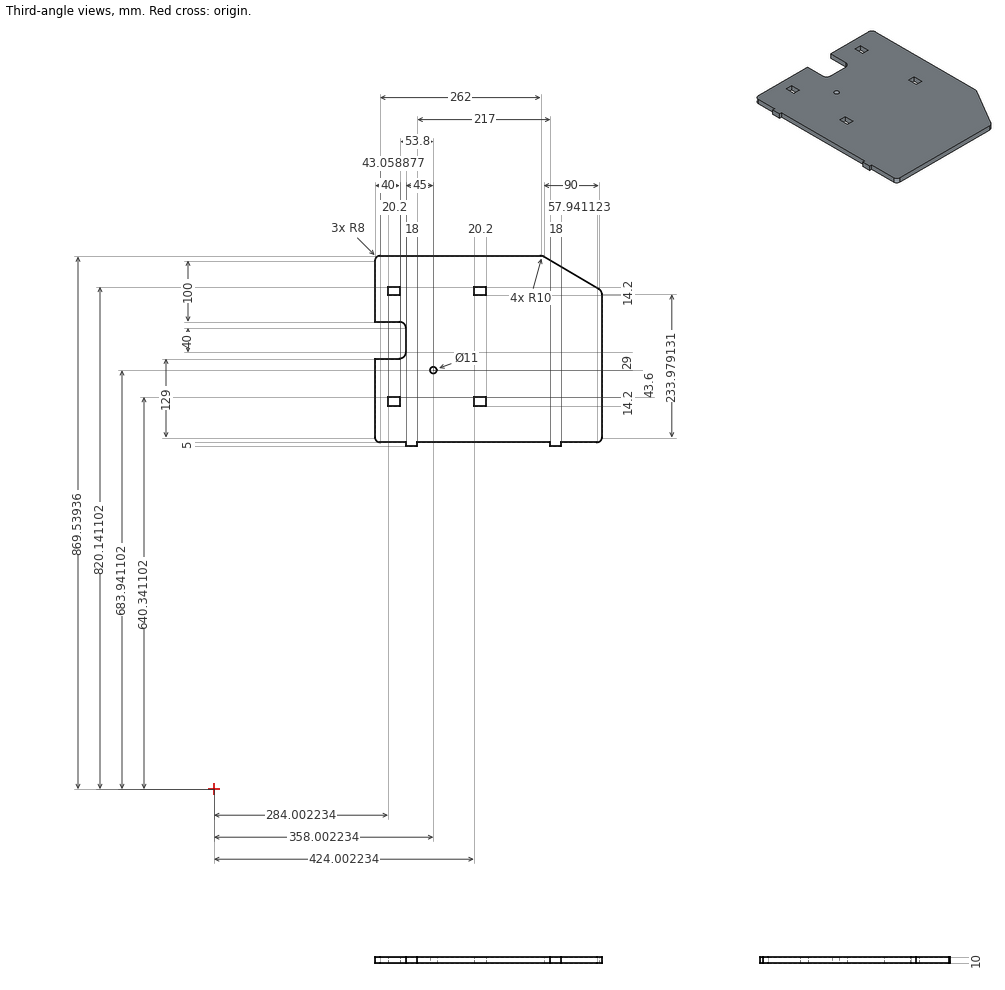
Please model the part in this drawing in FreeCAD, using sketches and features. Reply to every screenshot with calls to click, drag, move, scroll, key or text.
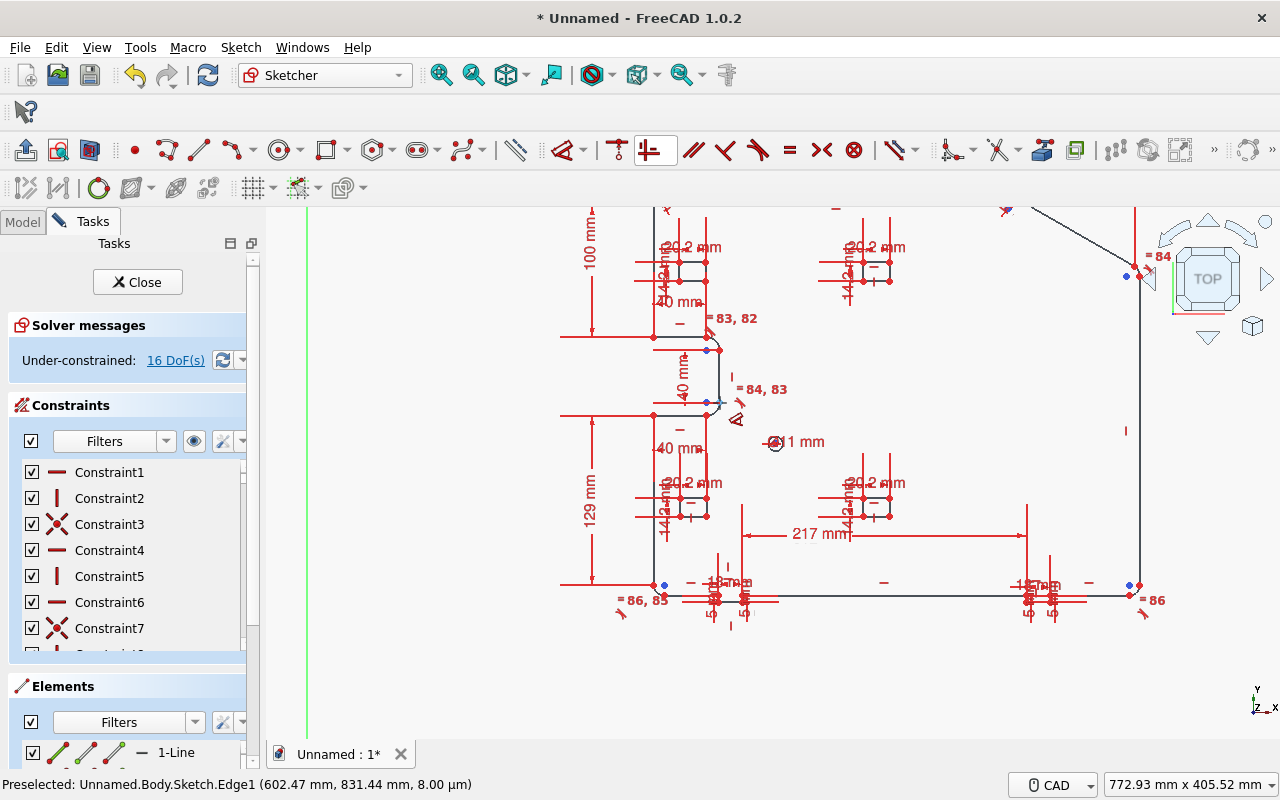
click(719, 403)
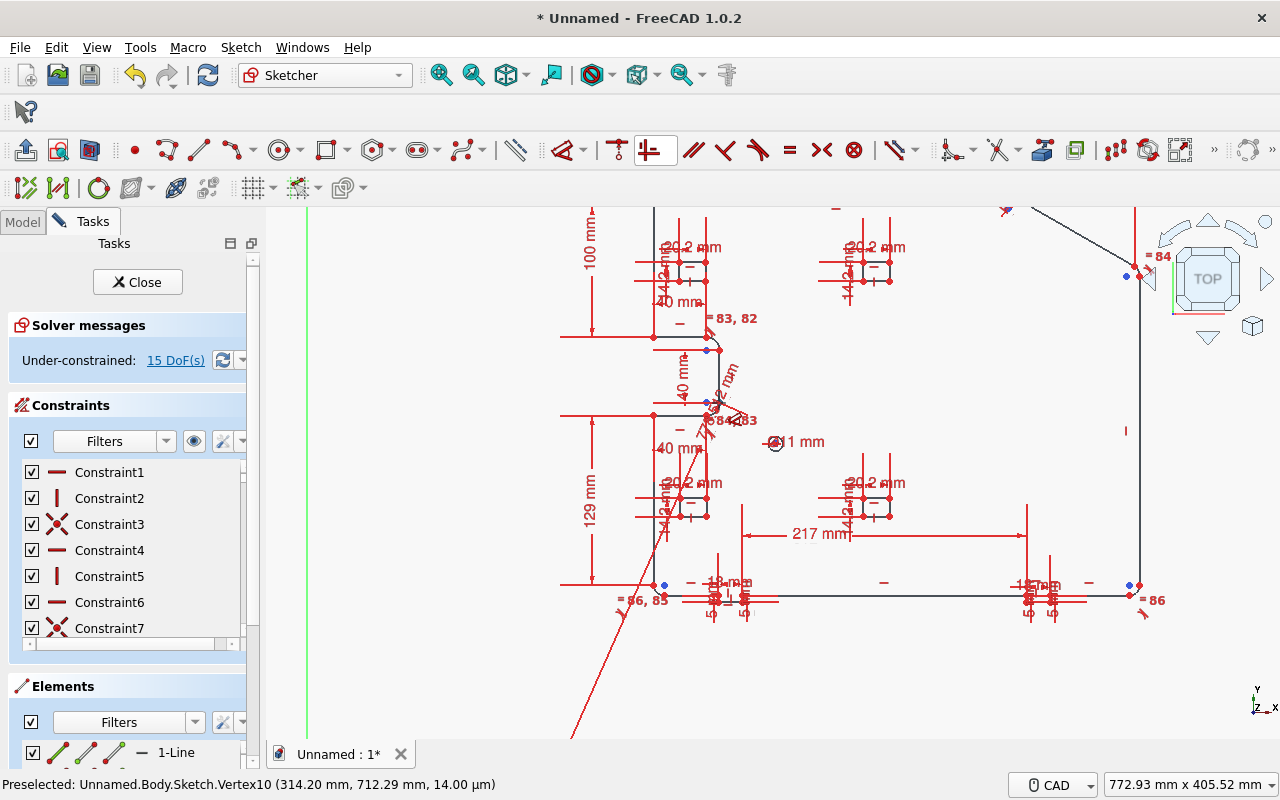
click(776, 444)
click(760, 369)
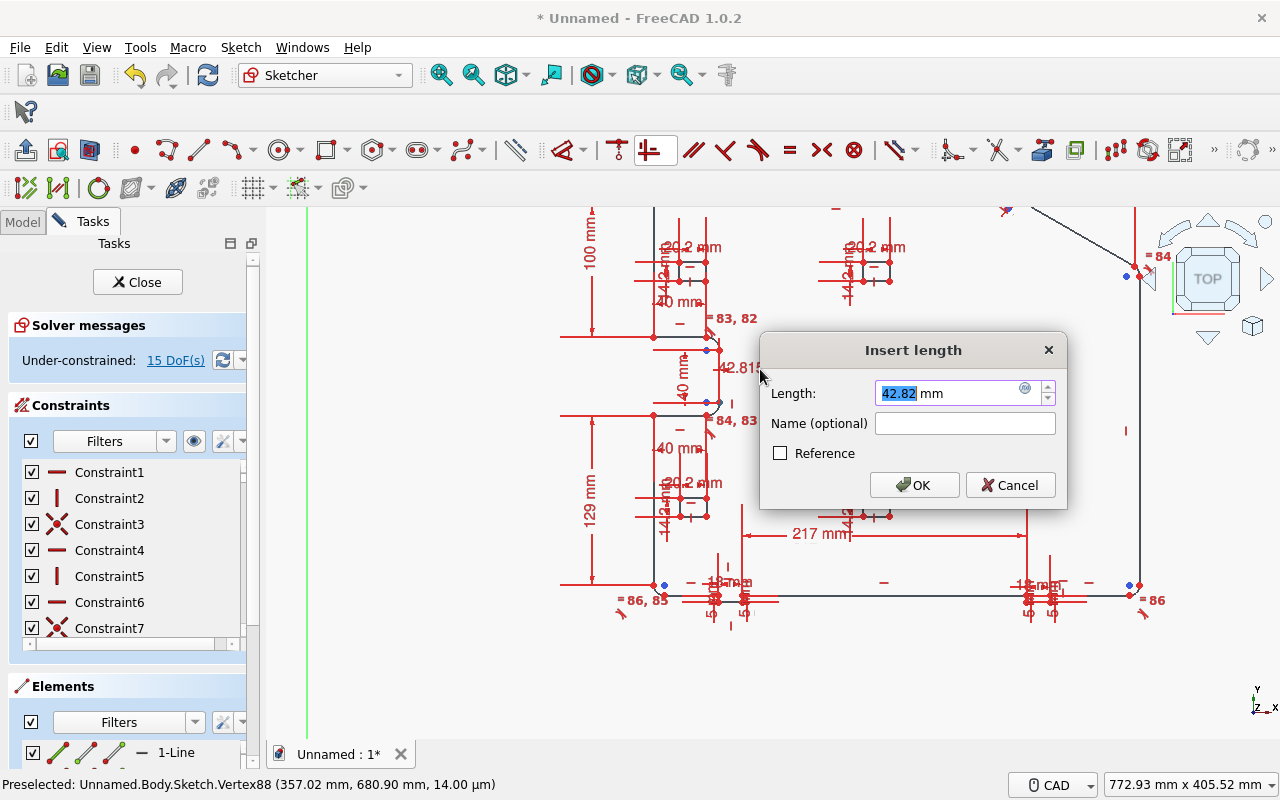
text(45)
key(Return)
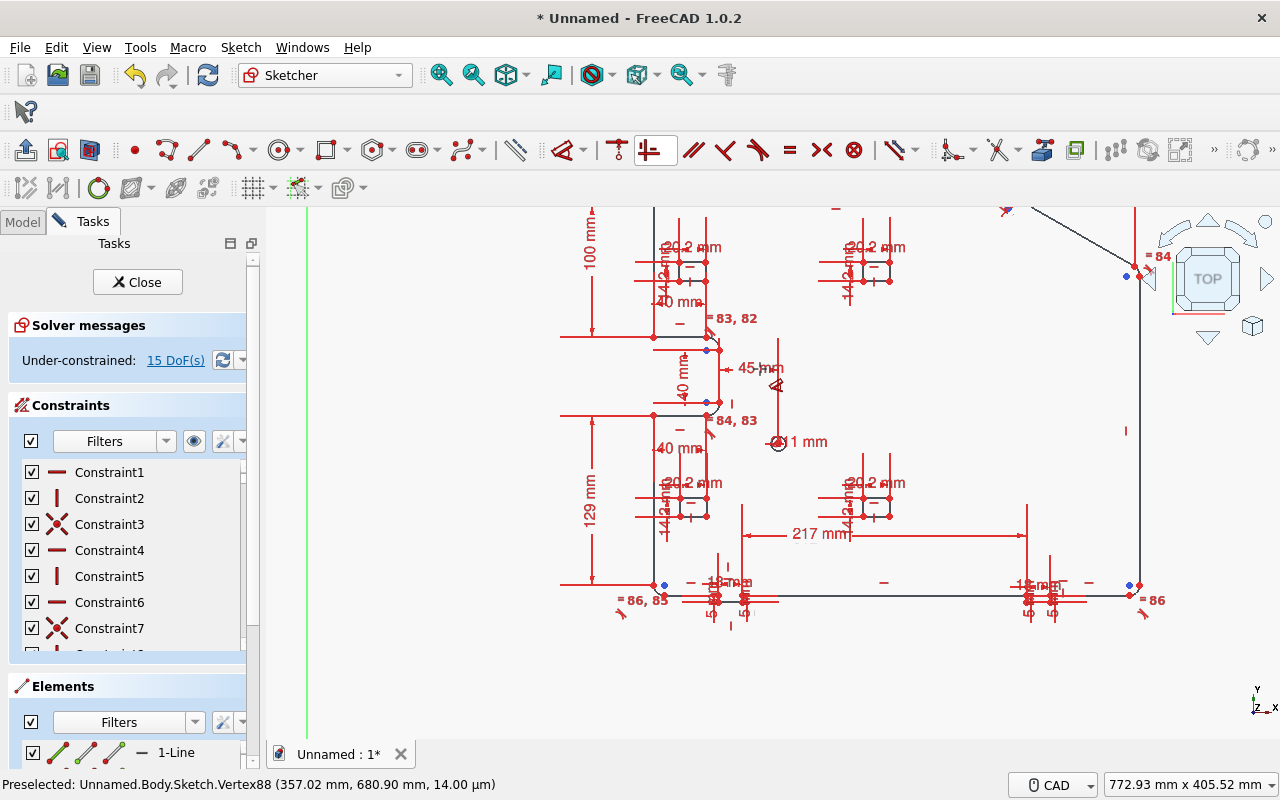
click(719, 403)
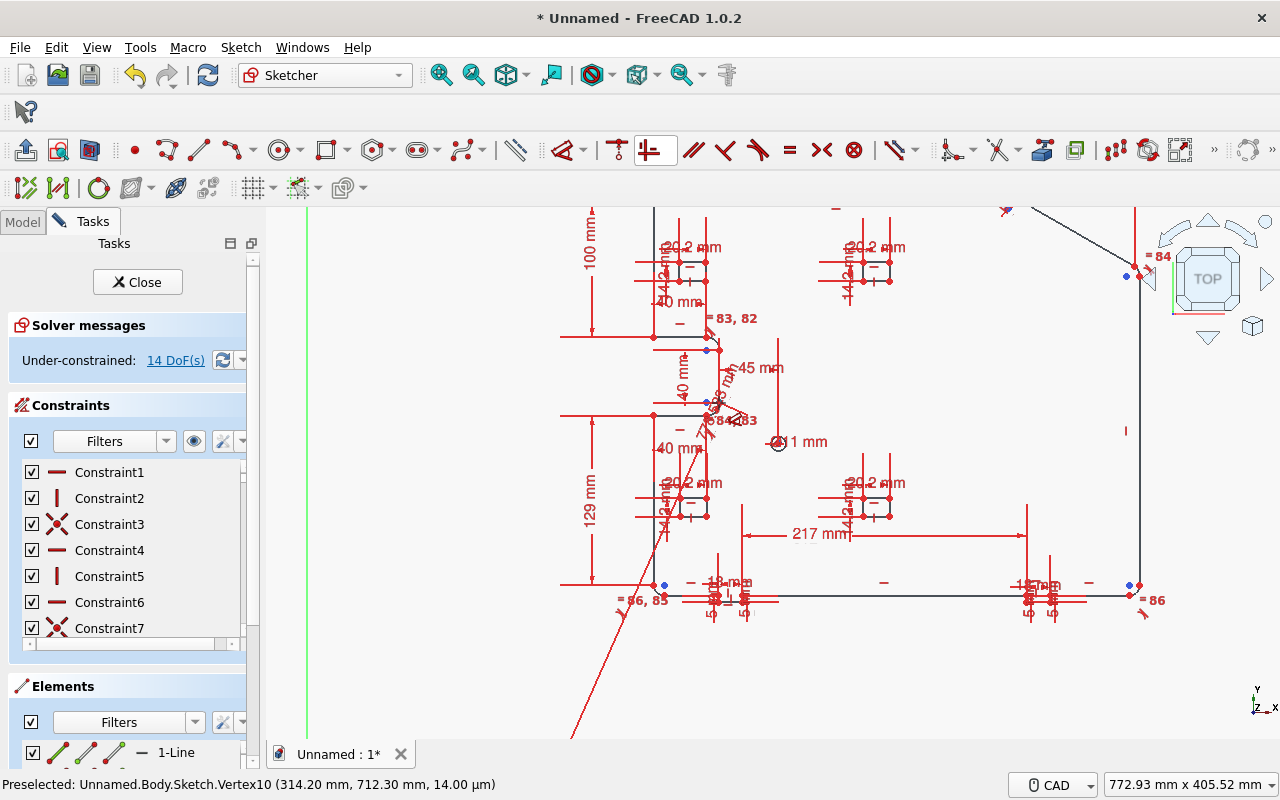
click(778, 444)
click(812, 423)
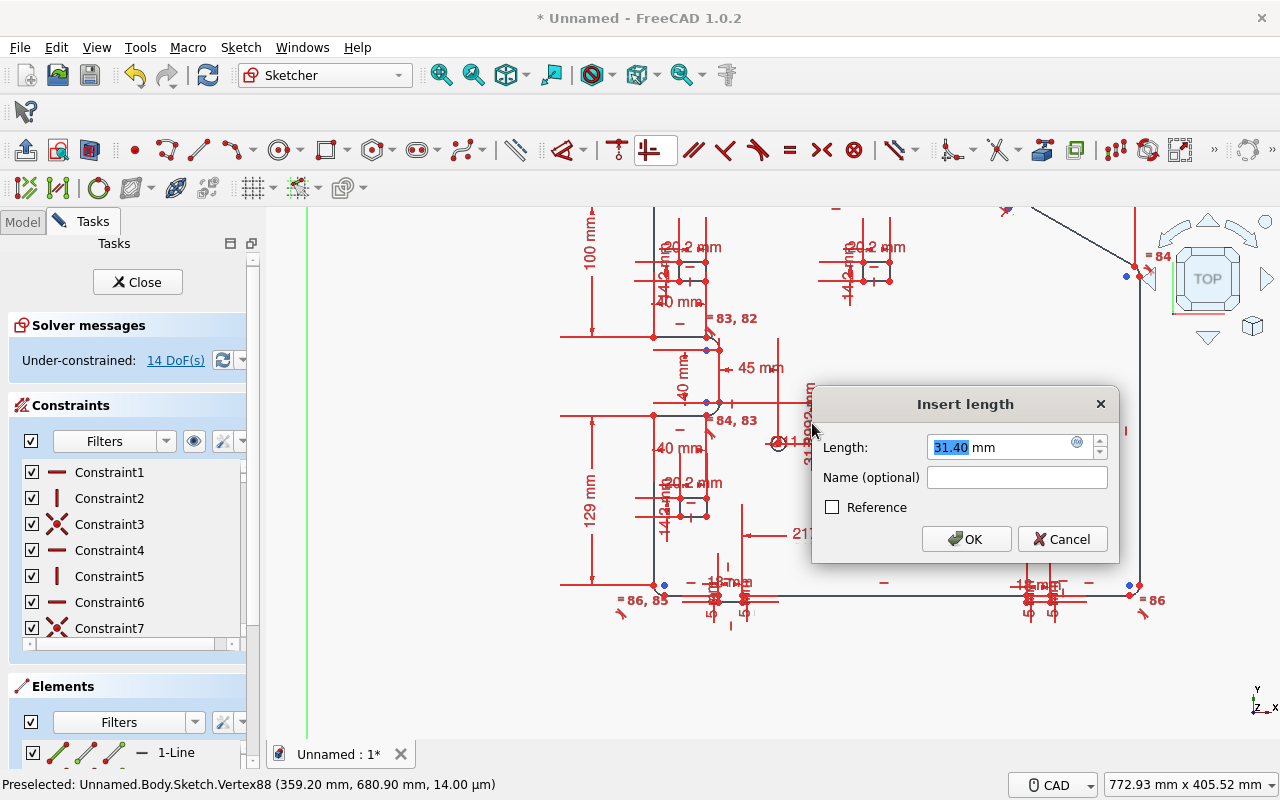
text(29)
key(Return)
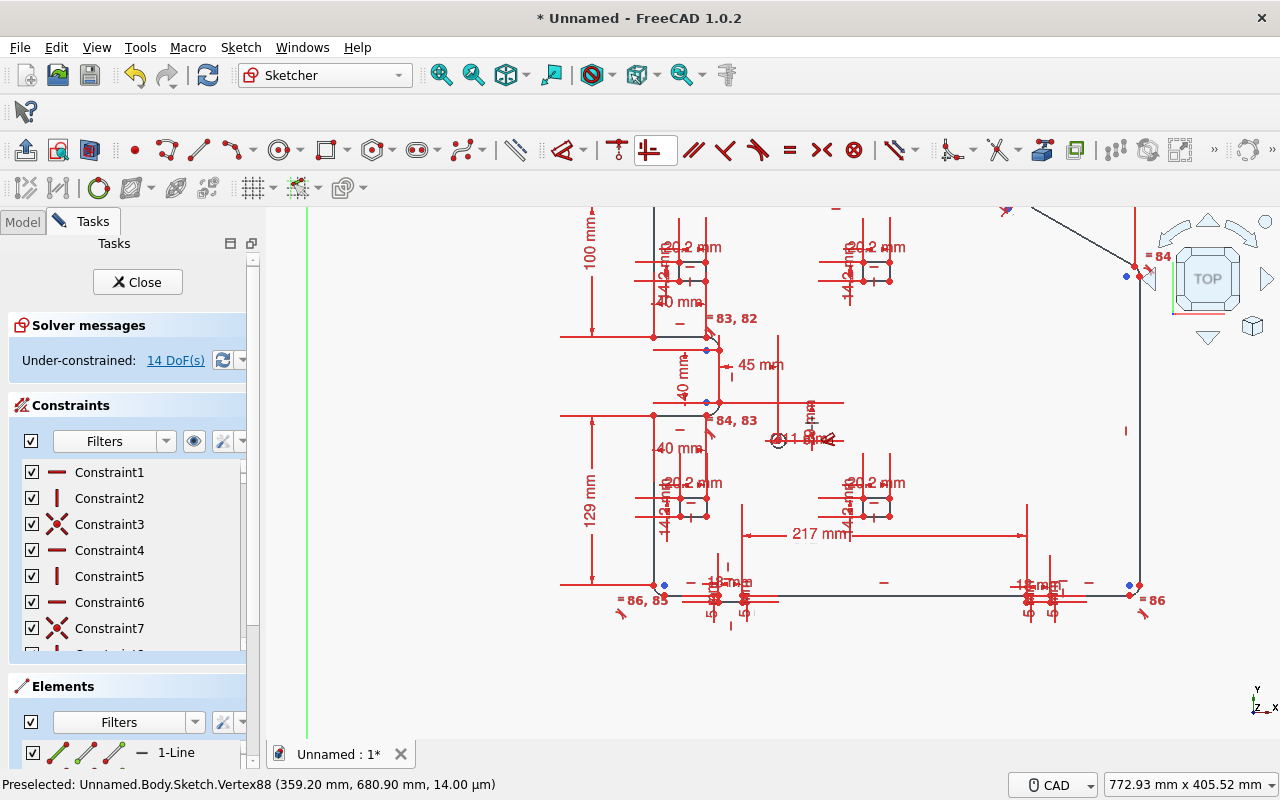
click(707, 498)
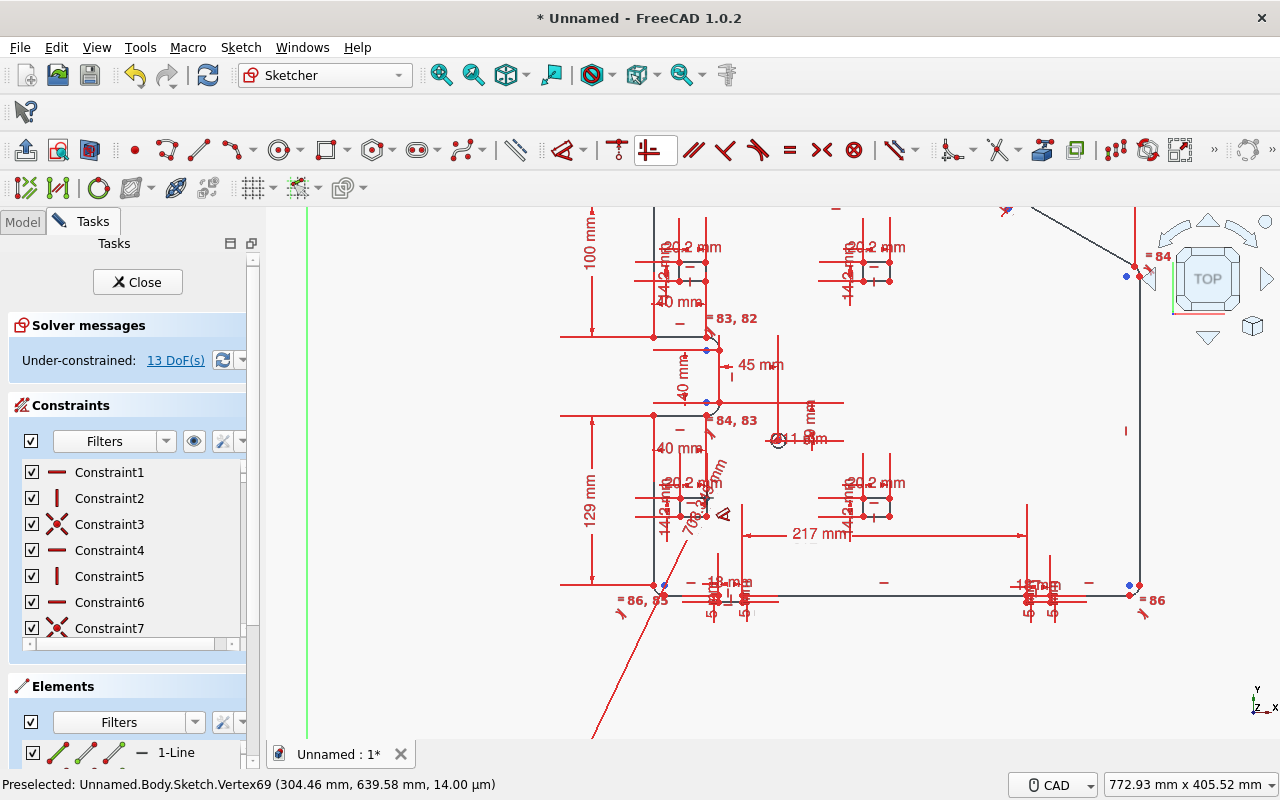
click(778, 441)
click(743, 532)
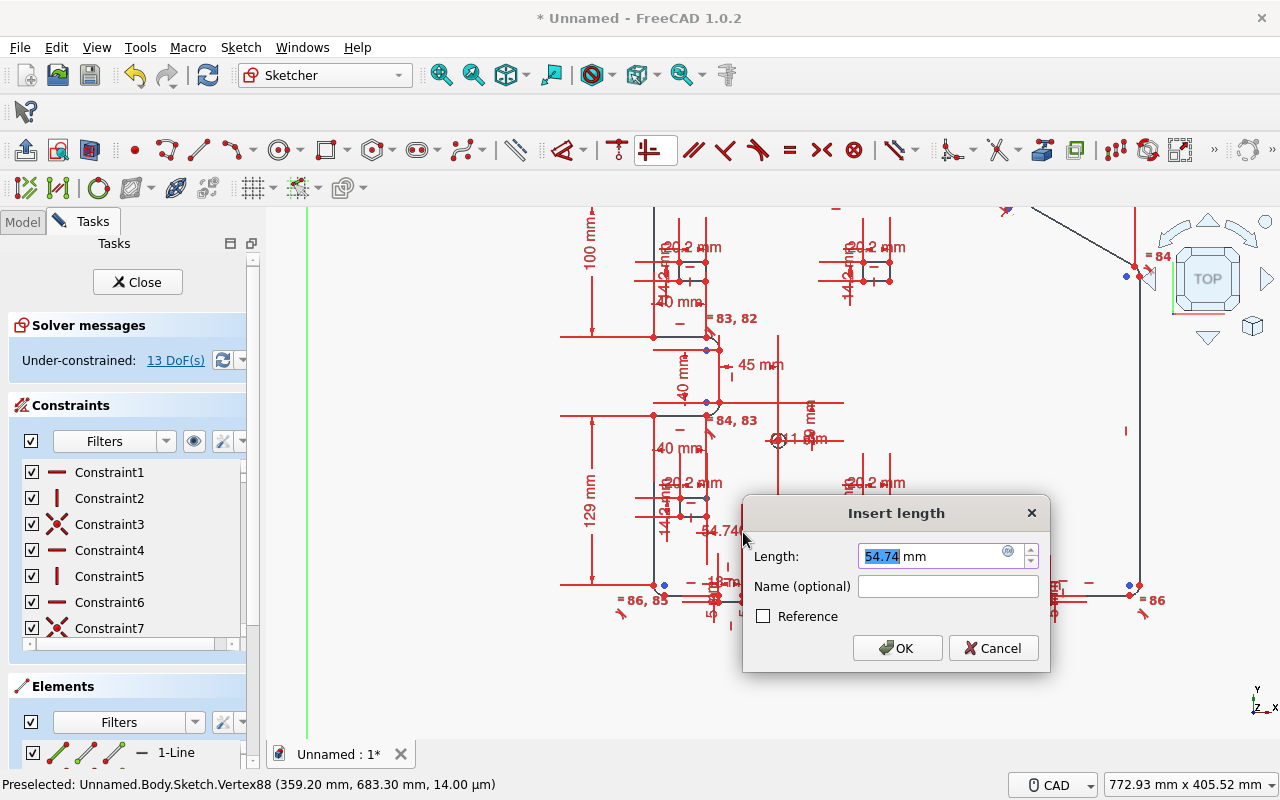
text(53.8)
key(Return)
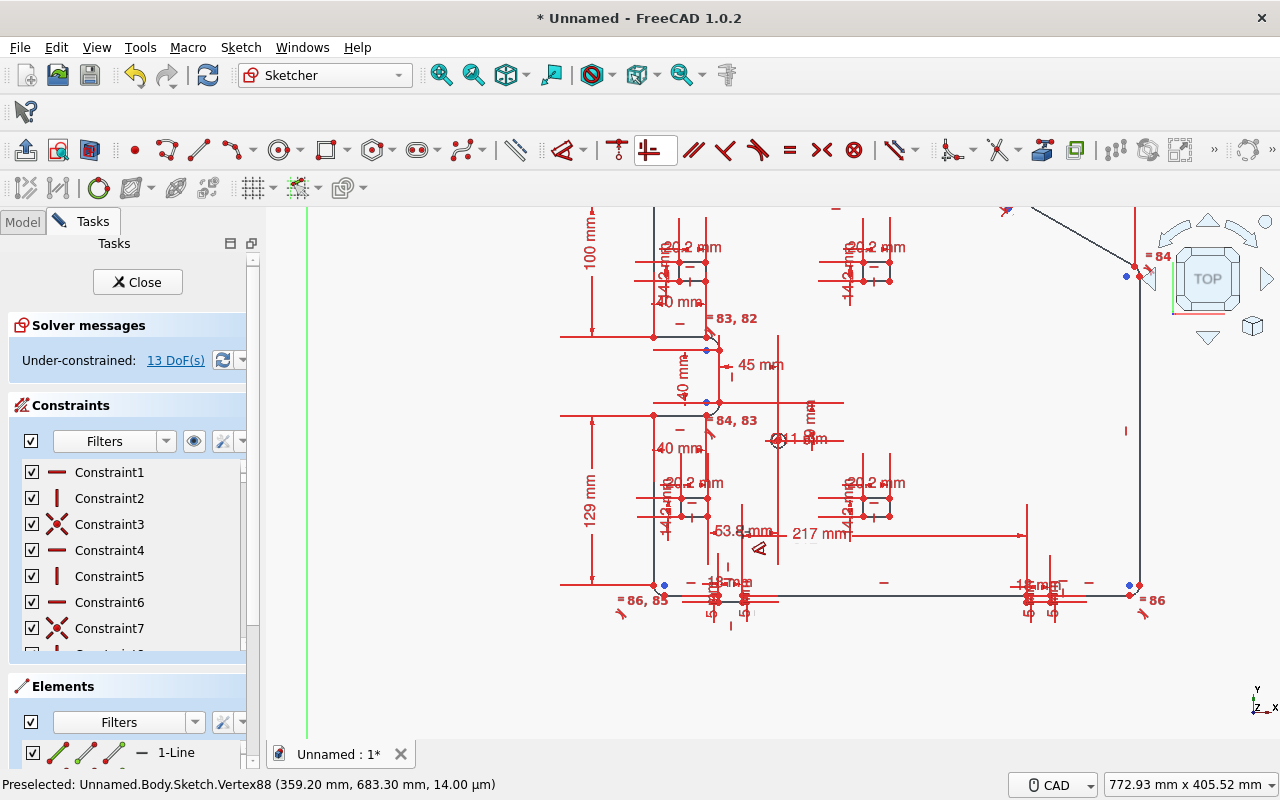
click(708, 498)